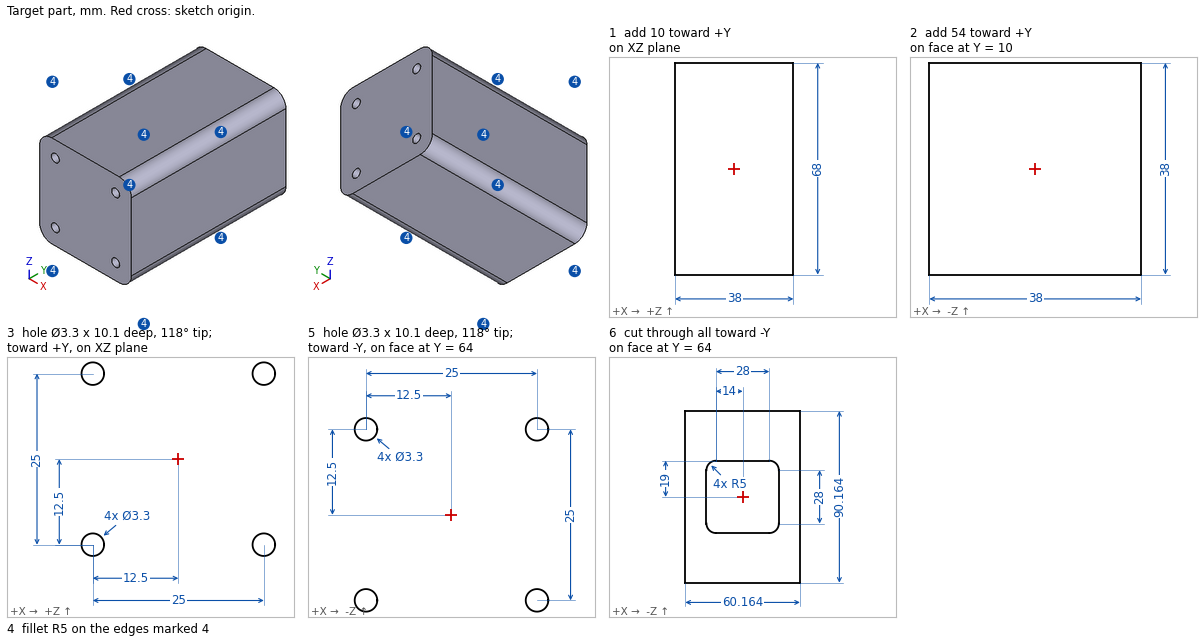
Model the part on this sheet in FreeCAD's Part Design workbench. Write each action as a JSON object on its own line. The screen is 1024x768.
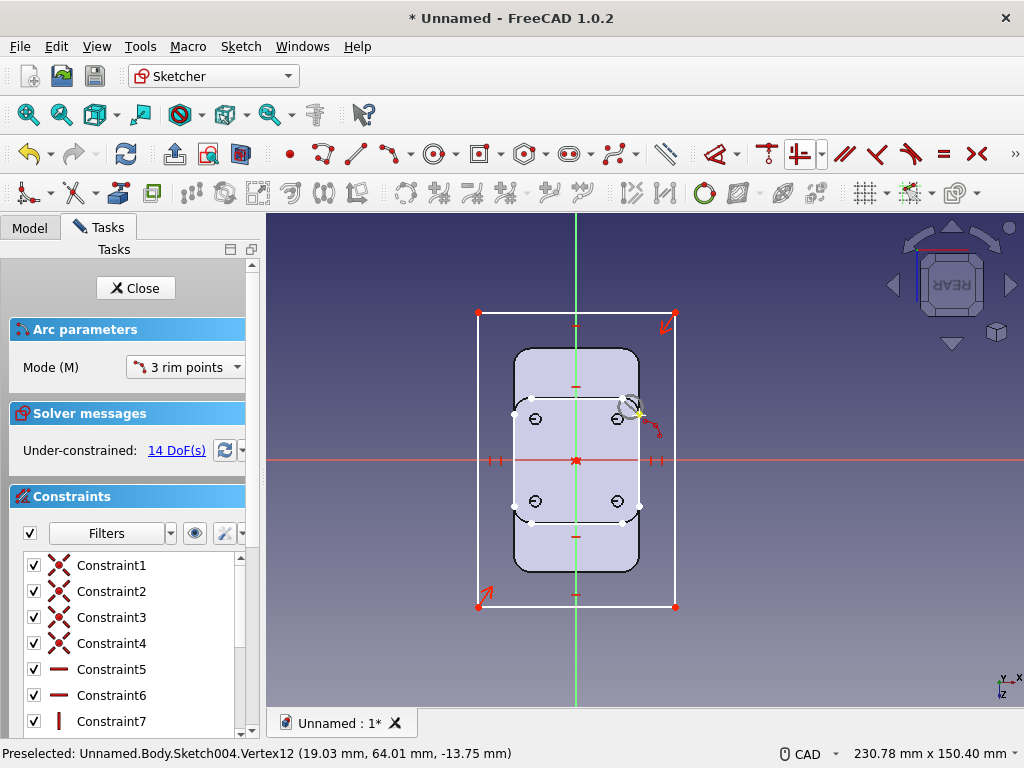
{"action": "scroll", "coordinate": [634, 403], "scroll_direction": "up", "scroll_amount": 6}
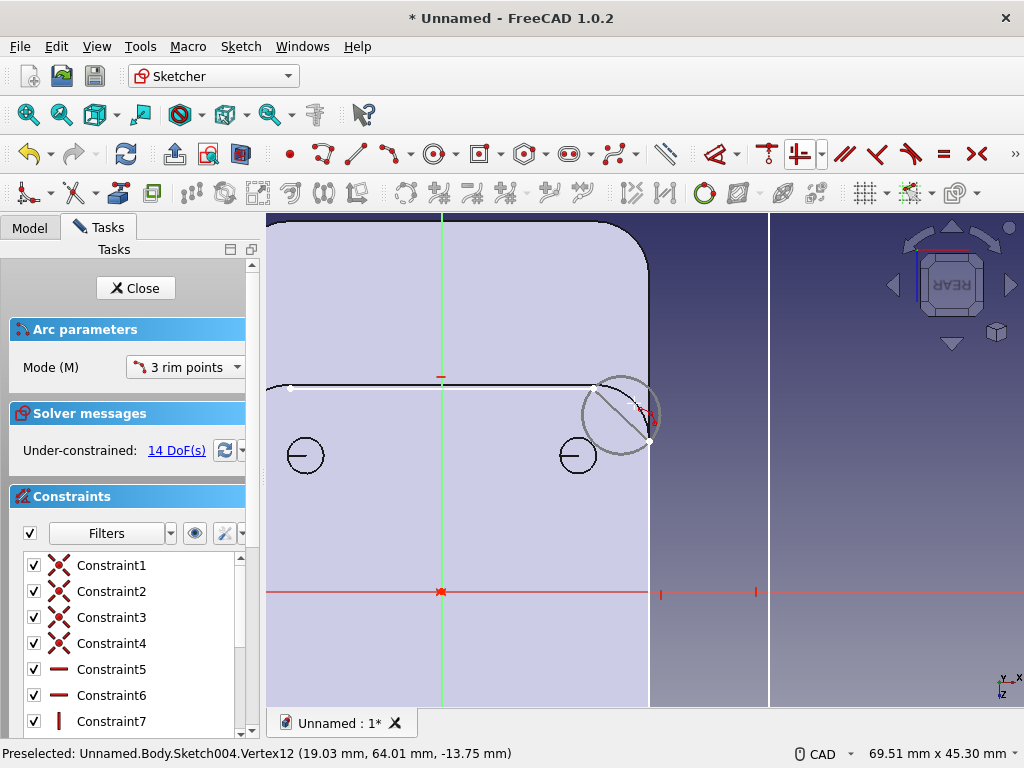
{"action": "left_click", "coordinate": [633, 401]}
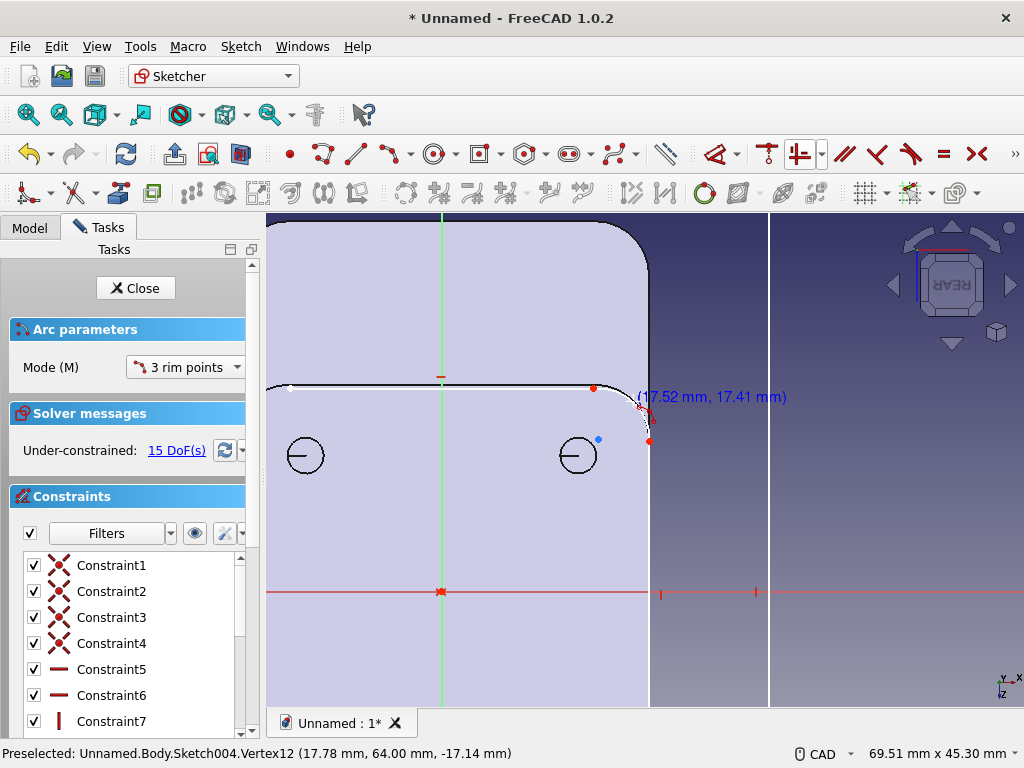
{"action": "scroll", "coordinate": [634, 403], "scroll_direction": "down", "scroll_amount": 6}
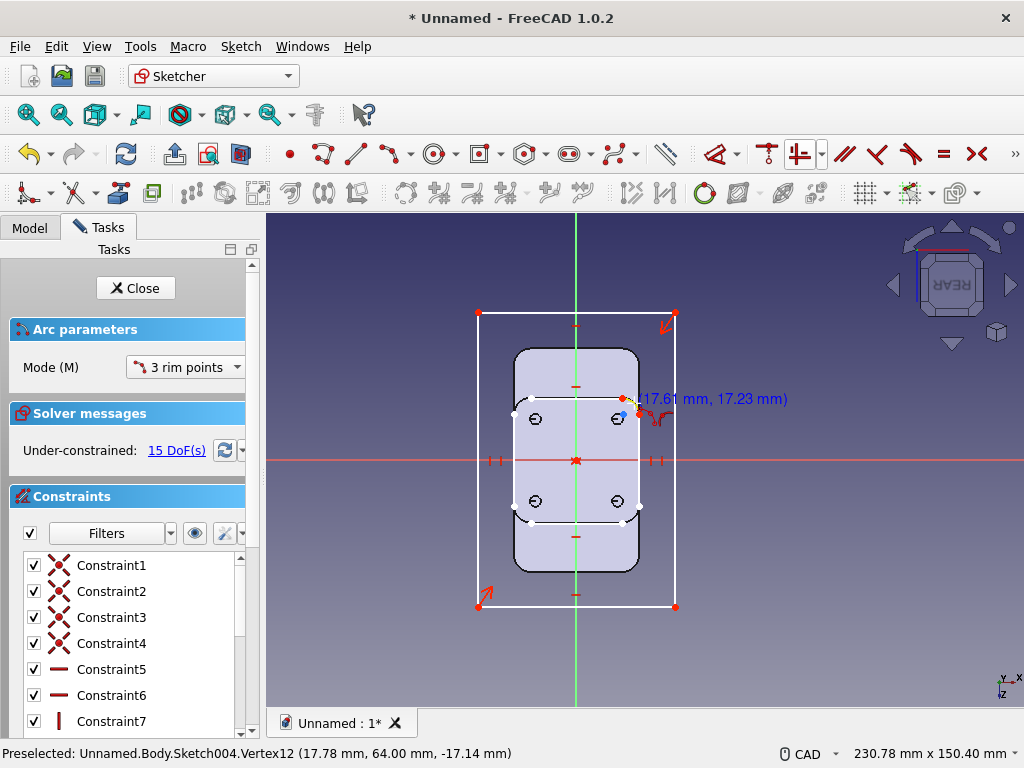
{"action": "left_click", "coordinate": [639, 507]}
{"action": "left_click", "coordinate": [622, 524]}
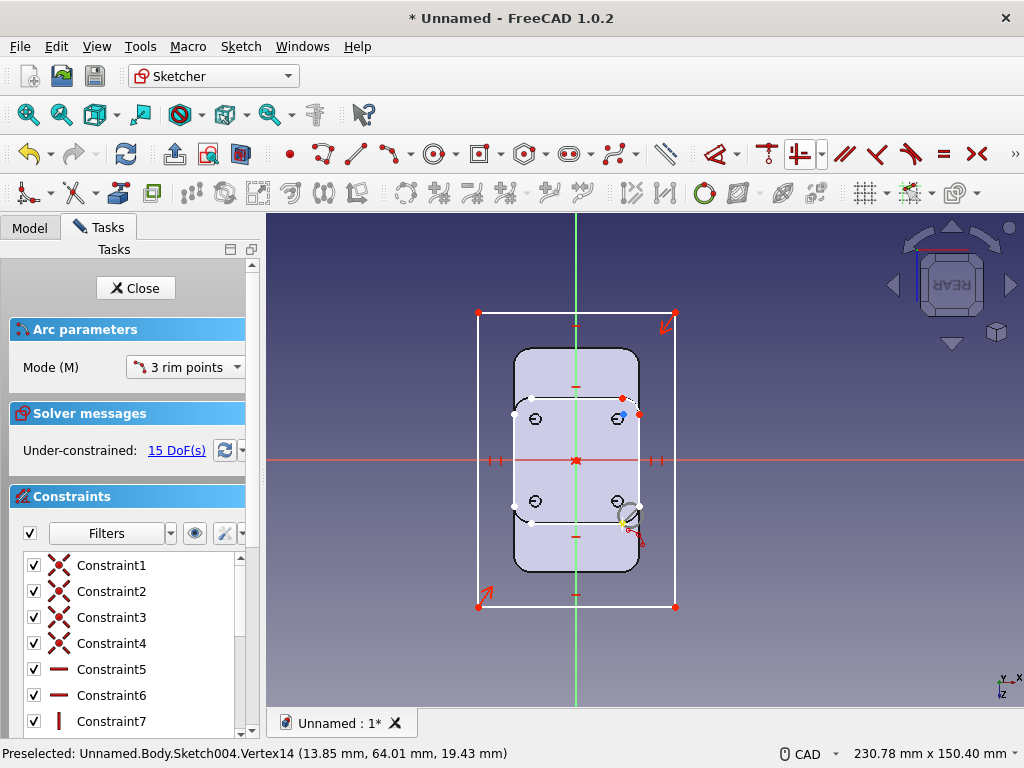
{"action": "scroll", "coordinate": [634, 518], "scroll_direction": "up", "scroll_amount": 6}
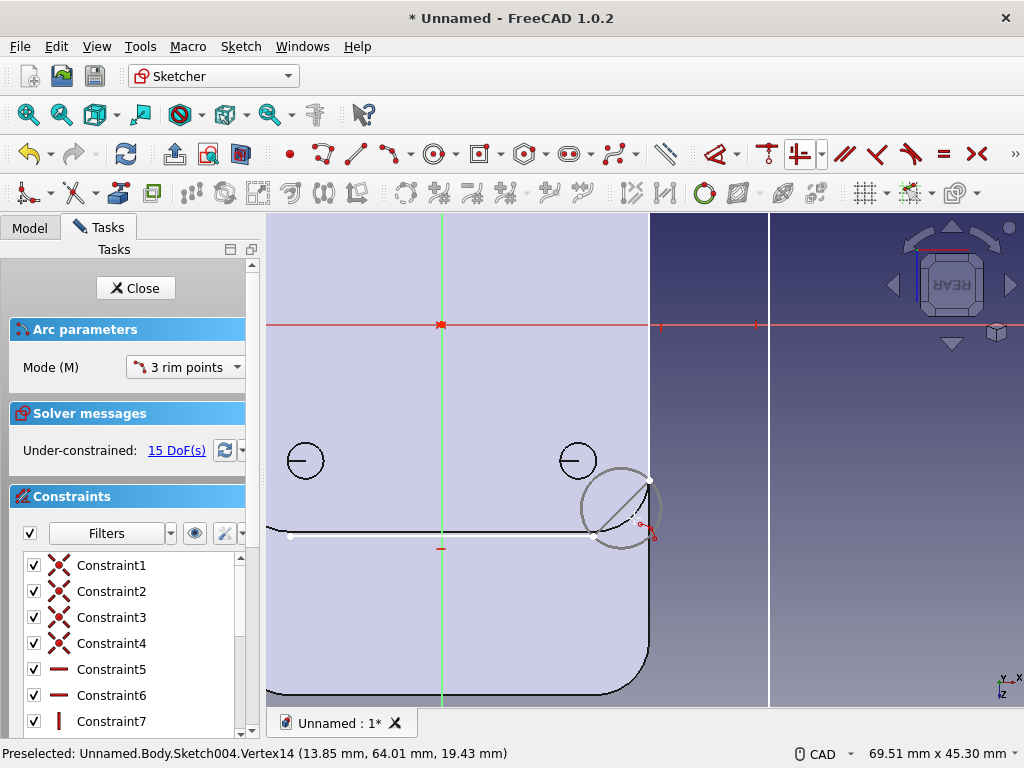
{"action": "left_click", "coordinate": [633, 516]}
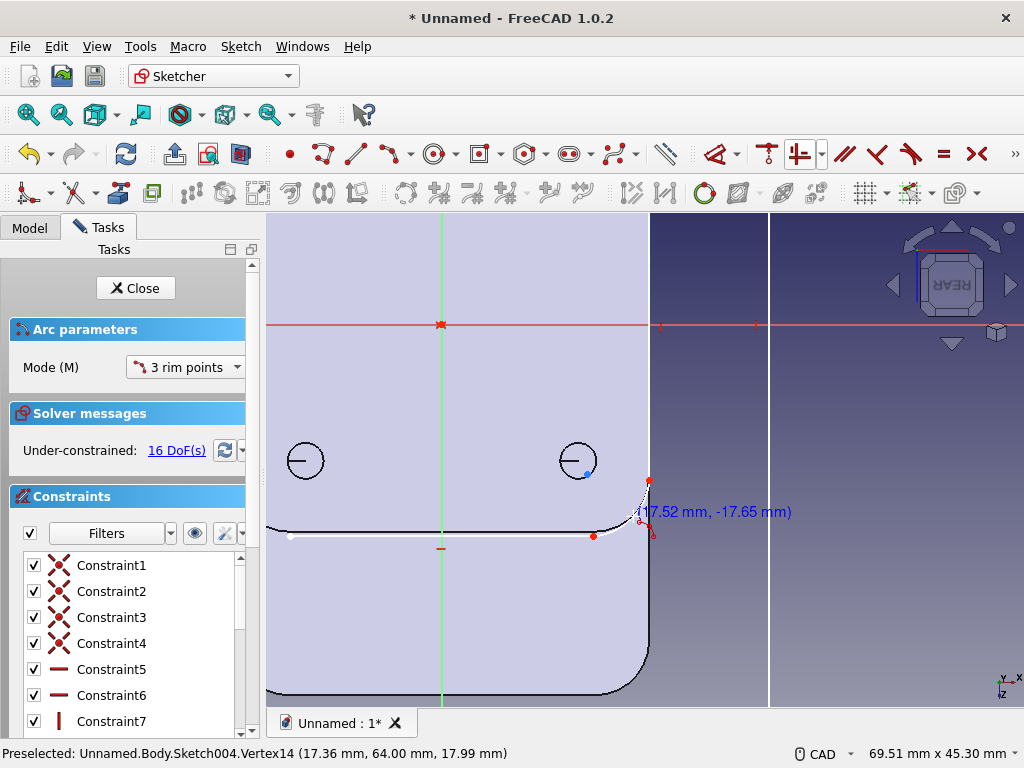
{"action": "scroll", "coordinate": [634, 518], "scroll_direction": "down", "scroll_amount": 6}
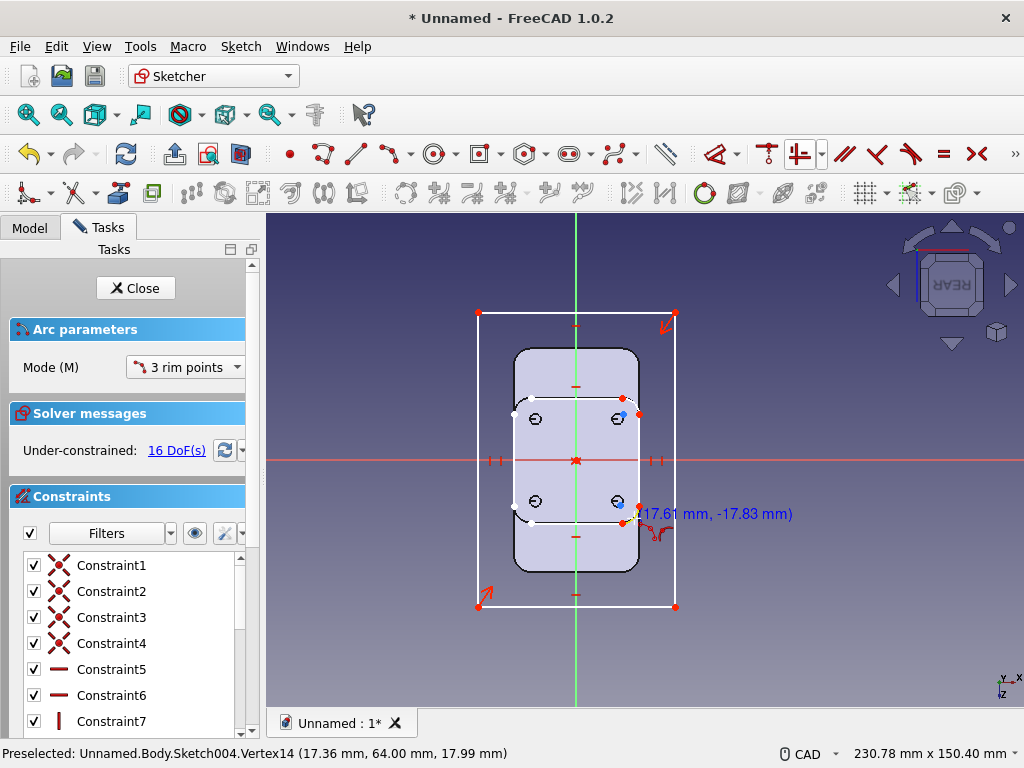
{"action": "left_click", "coordinate": [531, 524]}
{"action": "left_click", "coordinate": [514, 507]}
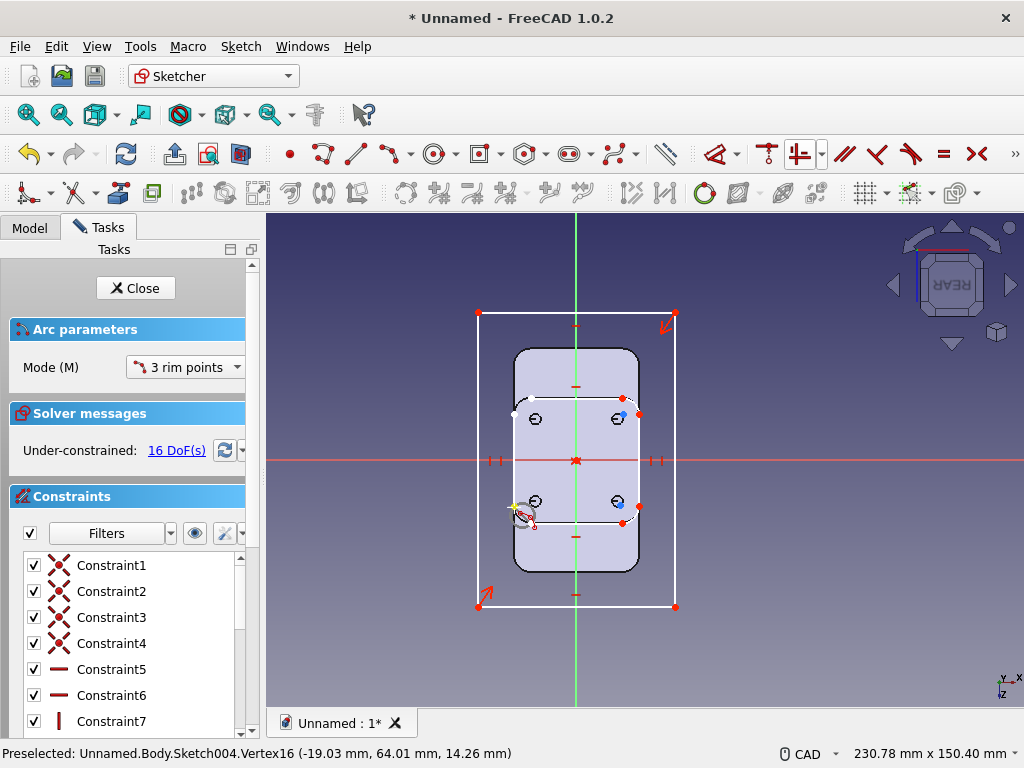
{"action": "scroll", "coordinate": [519, 518], "scroll_direction": "up", "scroll_amount": 6}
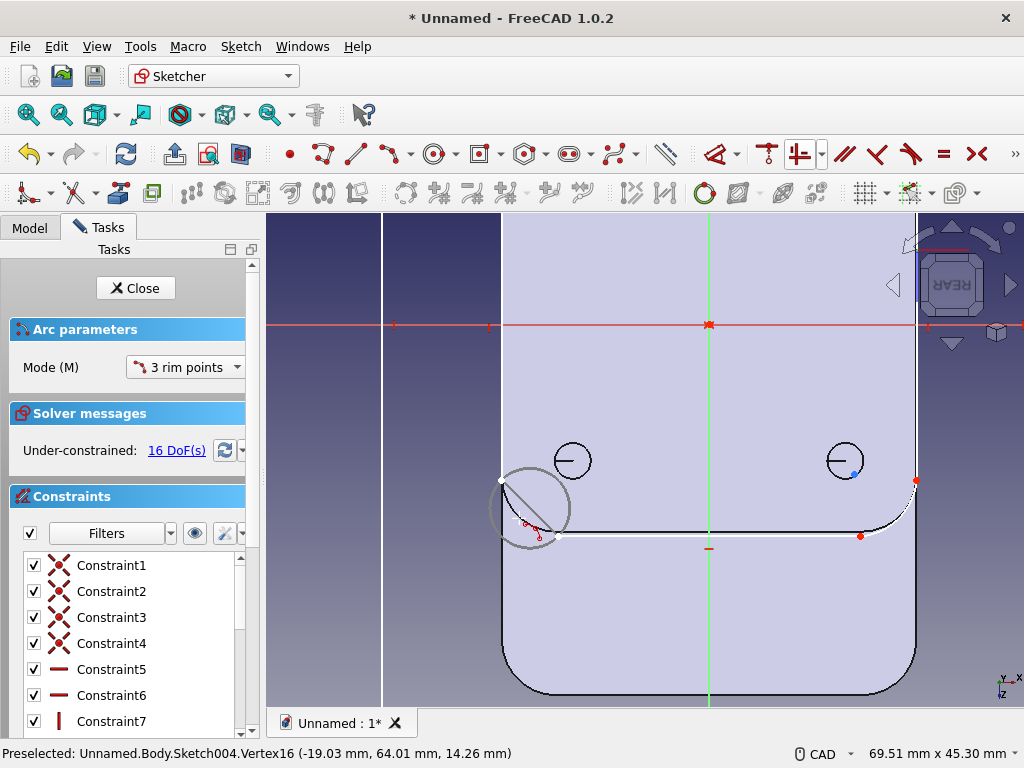
{"action": "left_click", "coordinate": [518, 516]}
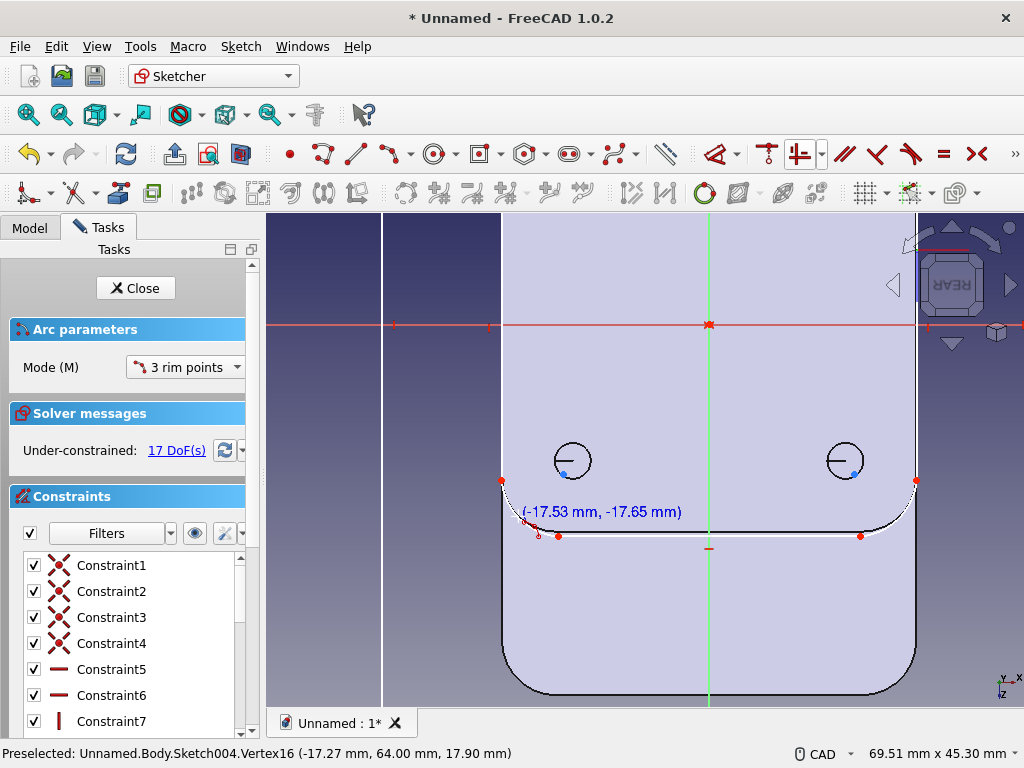
{"action": "scroll", "coordinate": [519, 518], "scroll_direction": "down", "scroll_amount": 6}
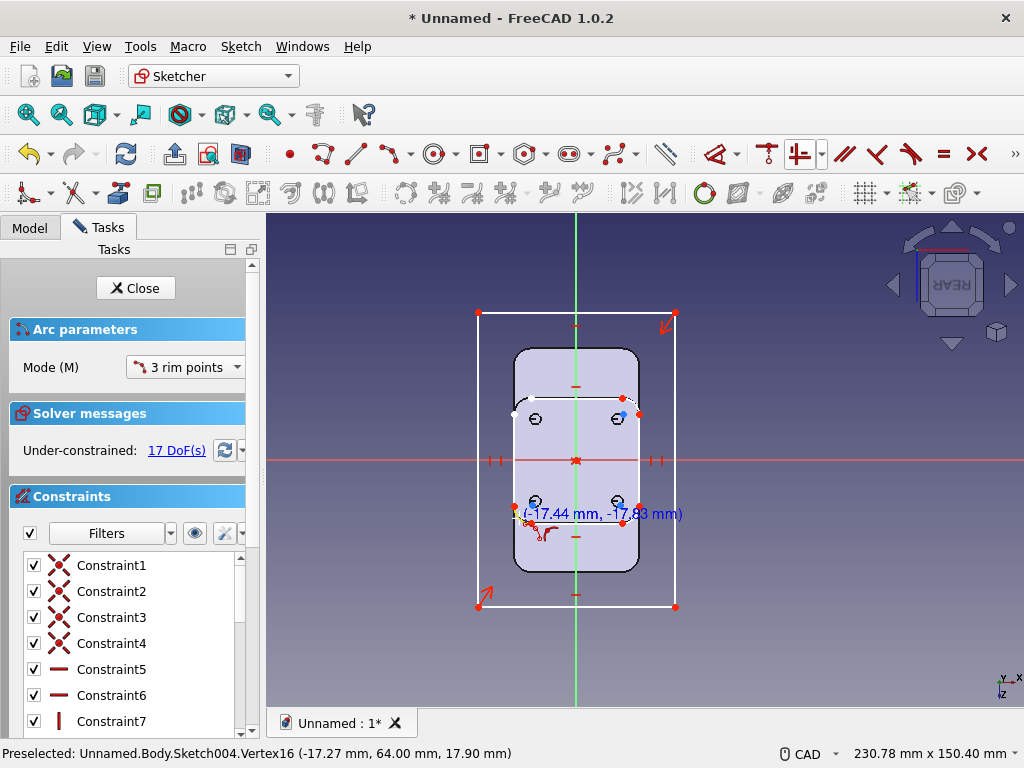
{"action": "left_click", "coordinate": [514, 415]}
{"action": "left_click", "coordinate": [531, 399]}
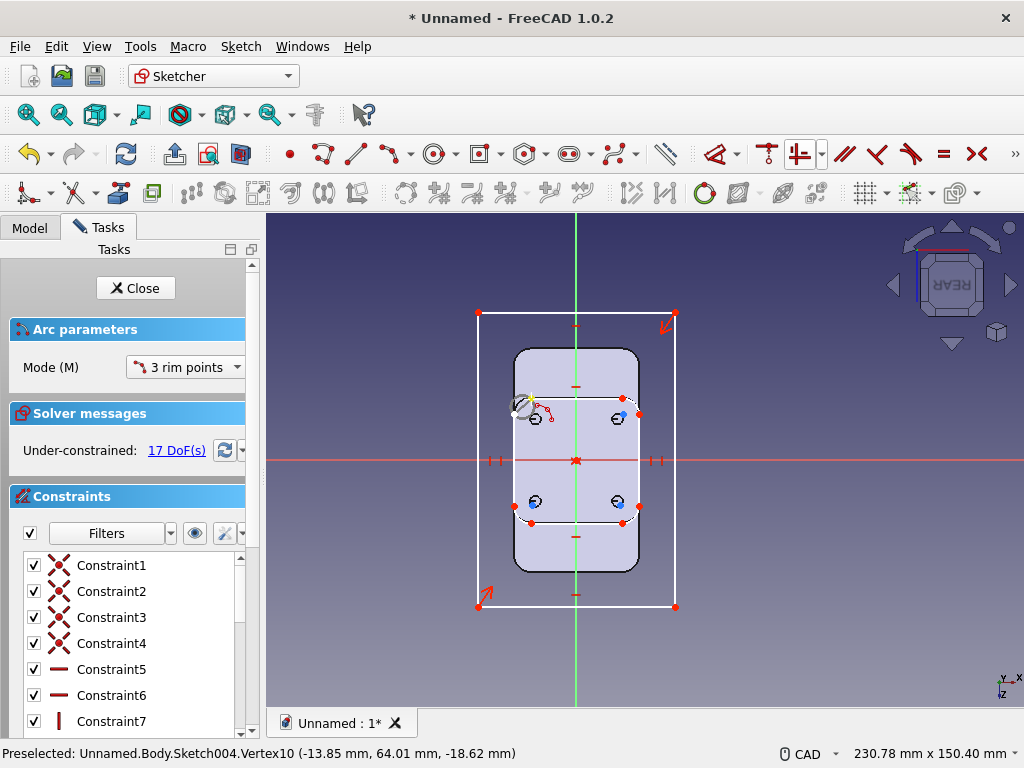
{"action": "scroll", "coordinate": [519, 403], "scroll_direction": "up", "scroll_amount": 6}